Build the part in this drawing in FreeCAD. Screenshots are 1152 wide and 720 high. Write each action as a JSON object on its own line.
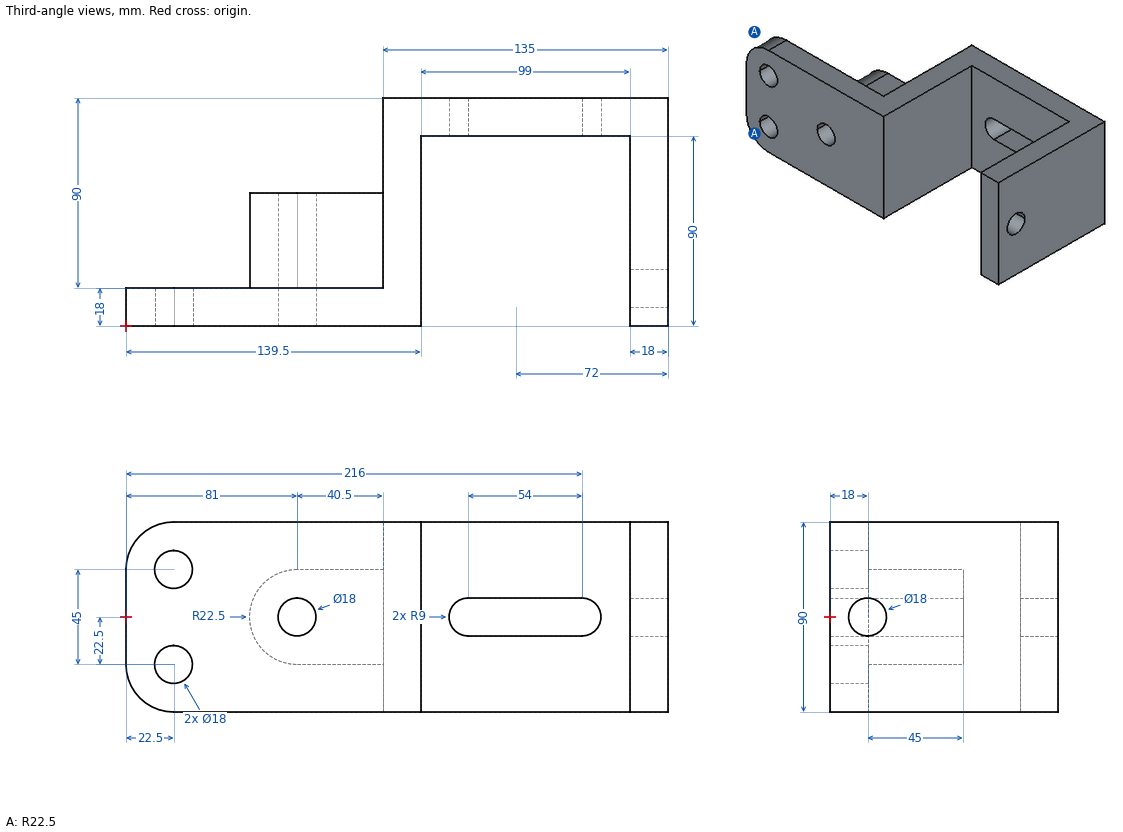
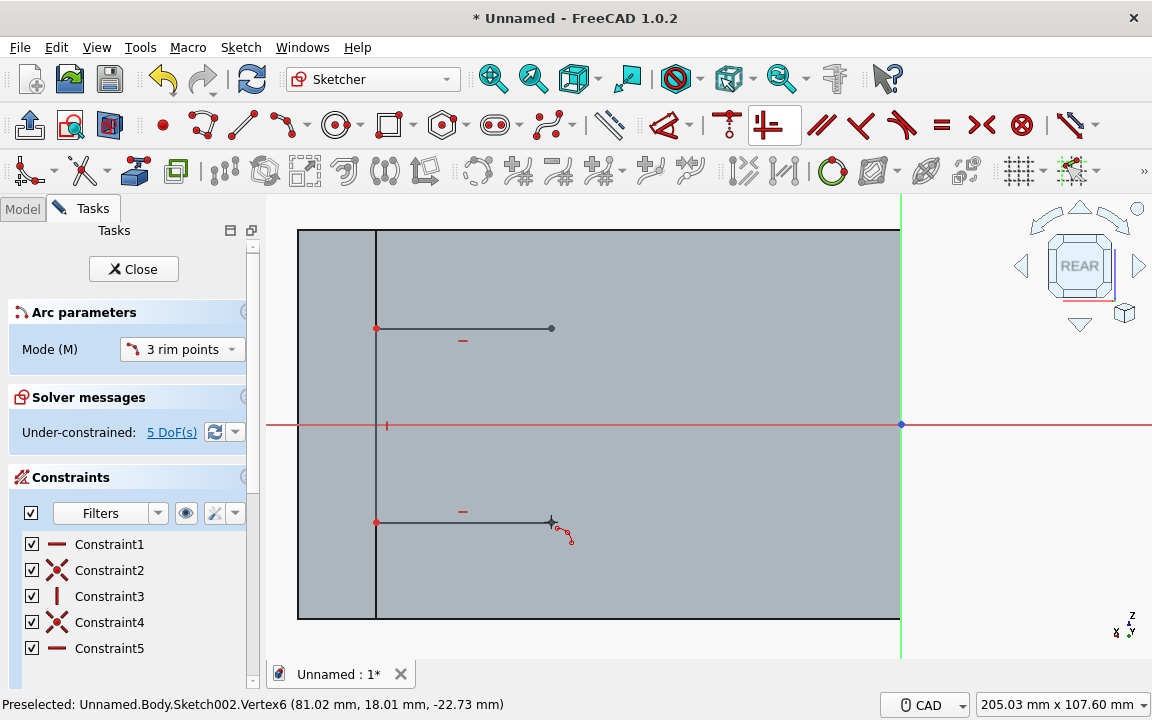
{"action": "left_click", "coordinate": [551, 523]}
{"action": "left_click", "coordinate": [551, 329]}
{"action": "left_click", "coordinate": [644, 455]}
{"action": "key", "text": "Escape"}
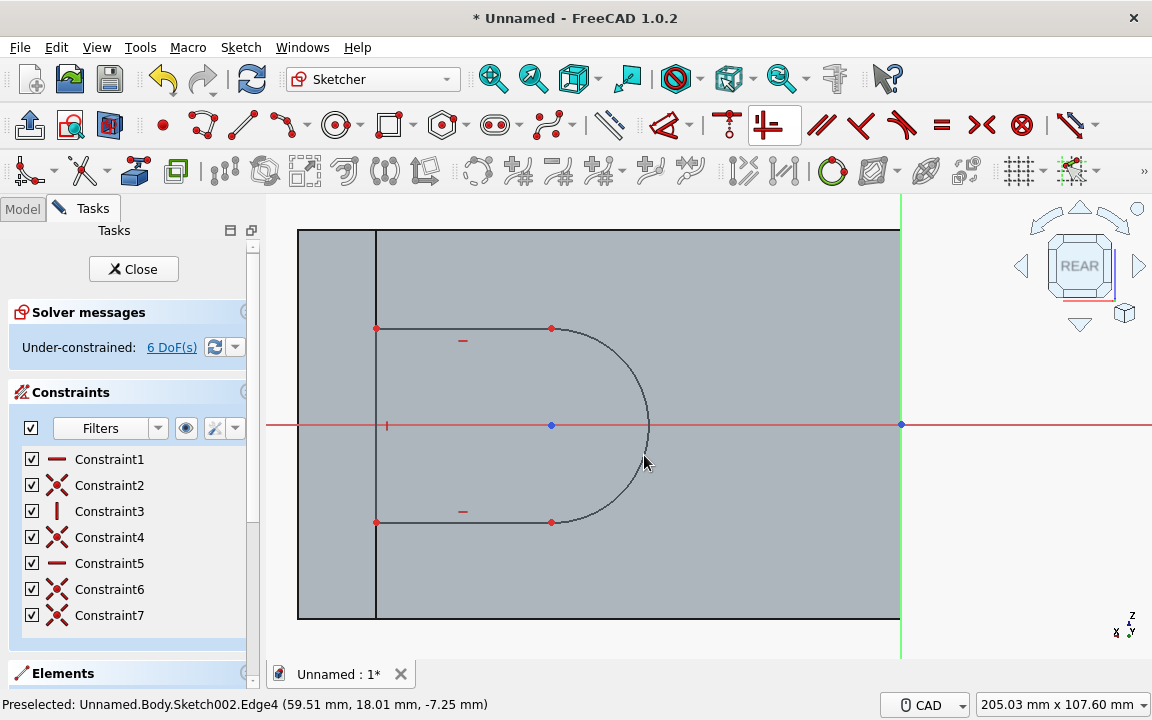
{"action": "left_click", "coordinate": [499, 329]}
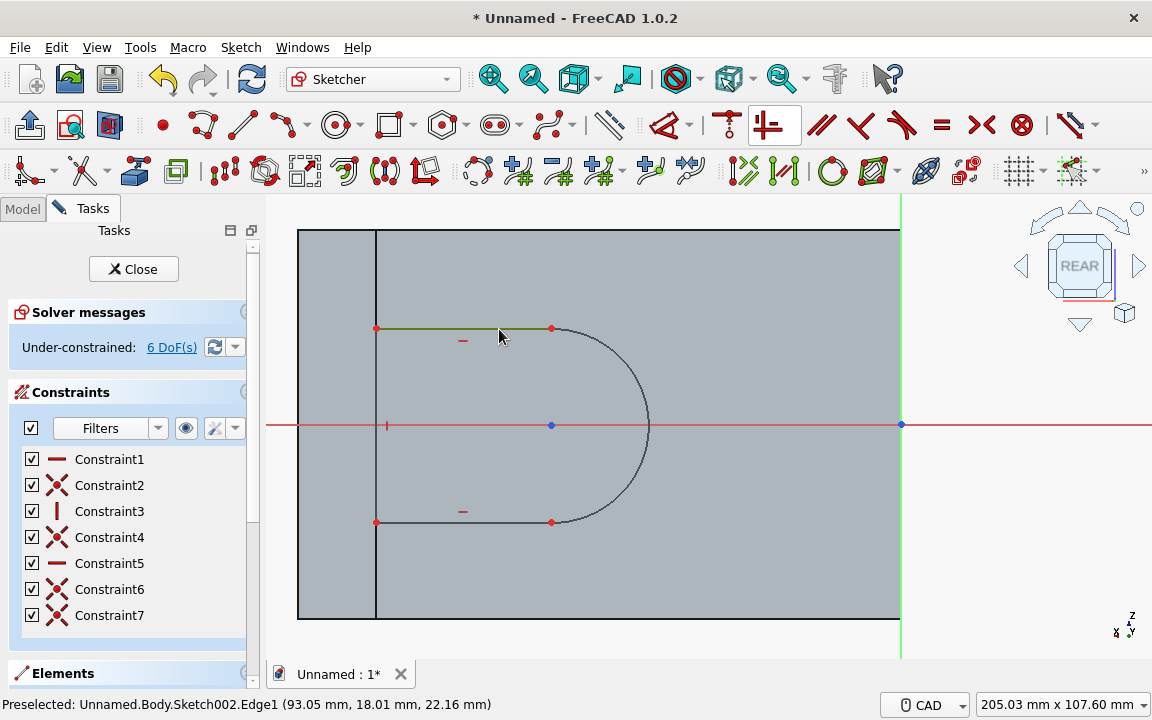
{"action": "left_click", "coordinate": [630, 483]}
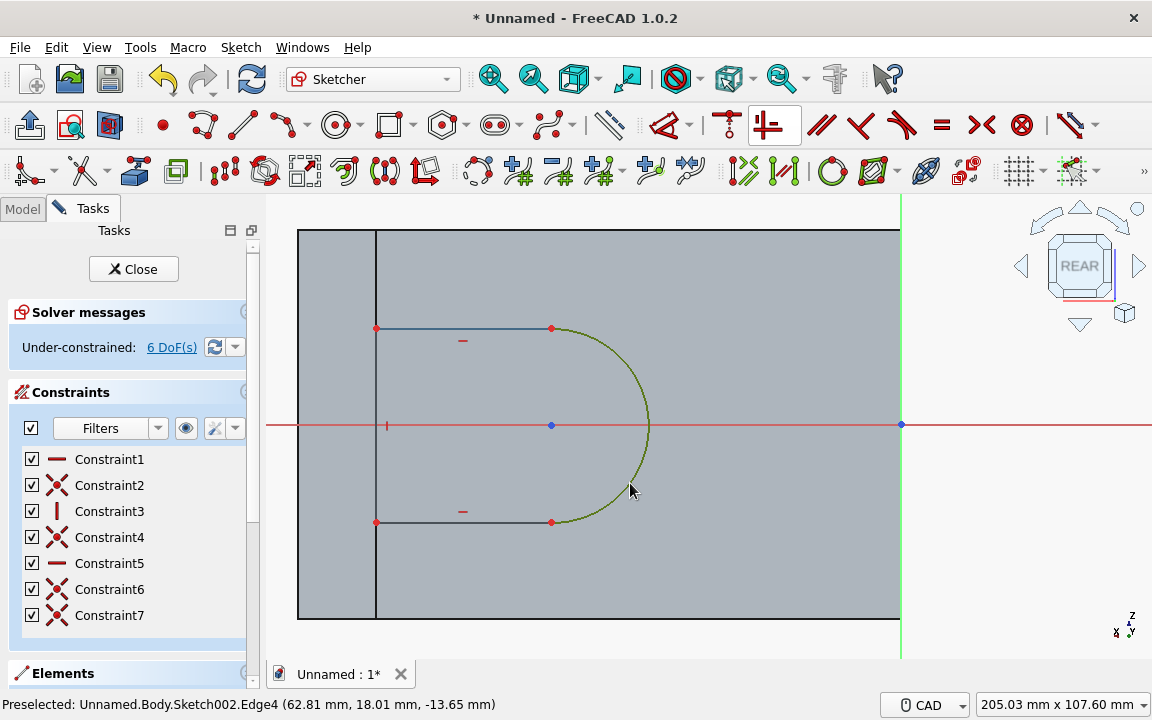
{"action": "left_click", "coordinate": [902, 126]}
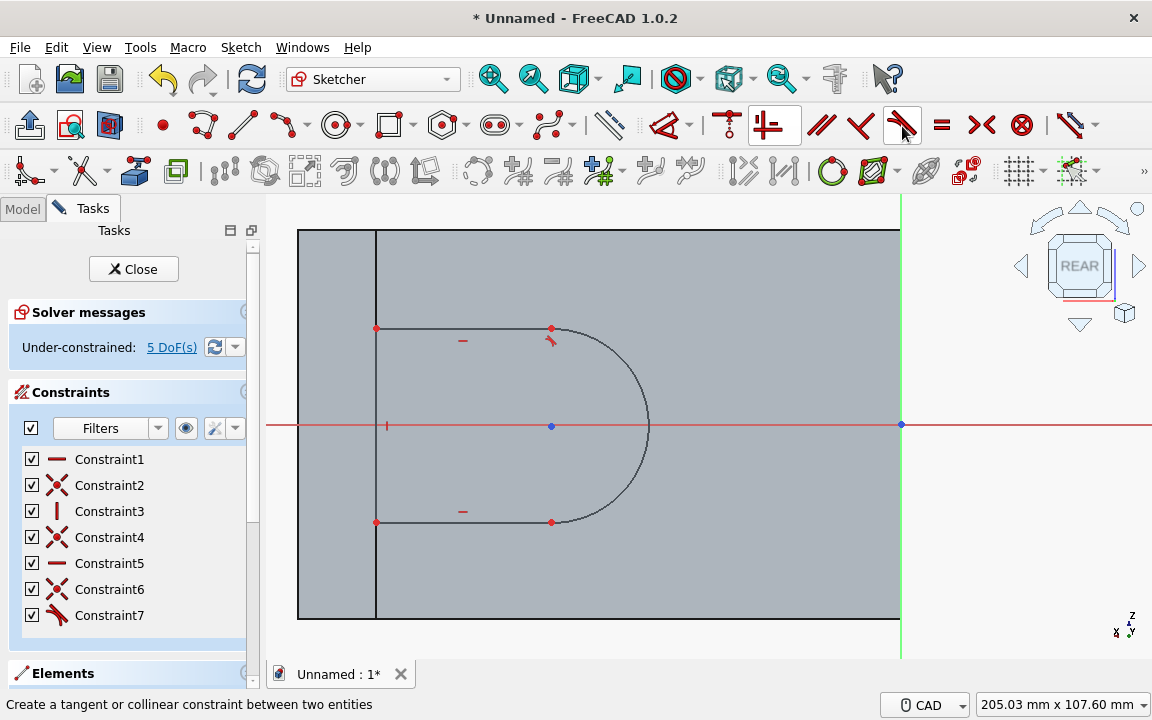
{"action": "left_click", "coordinate": [429, 523]}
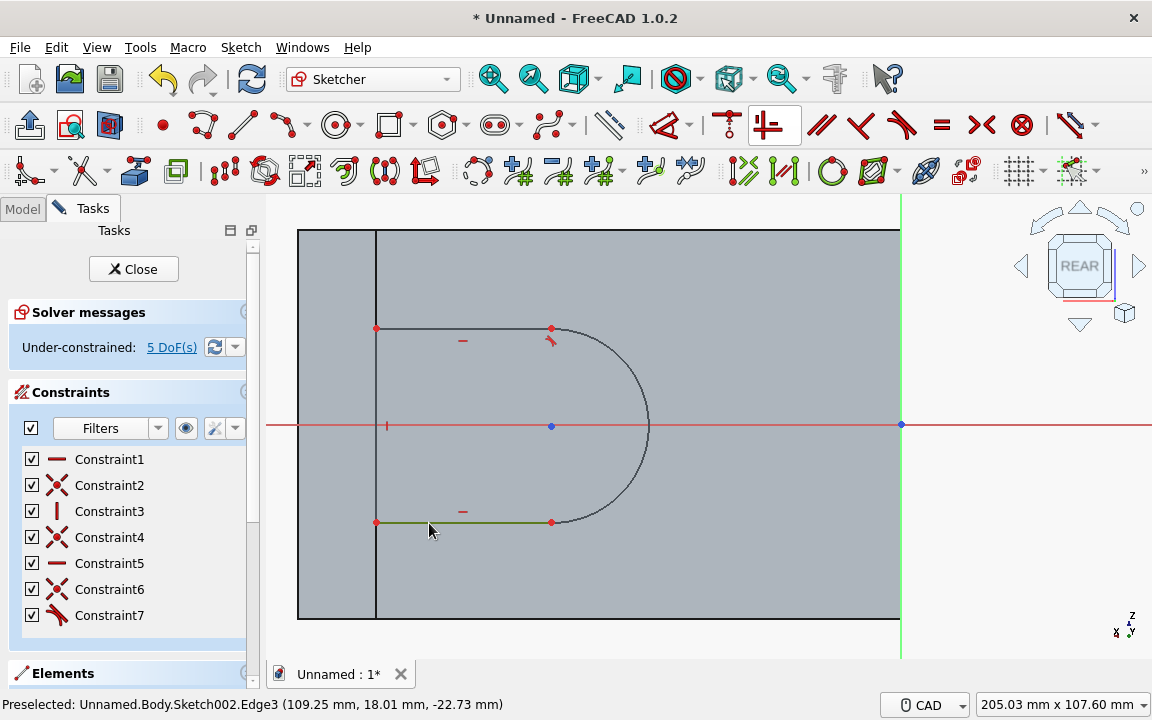
{"action": "left_click", "coordinate": [630, 483]}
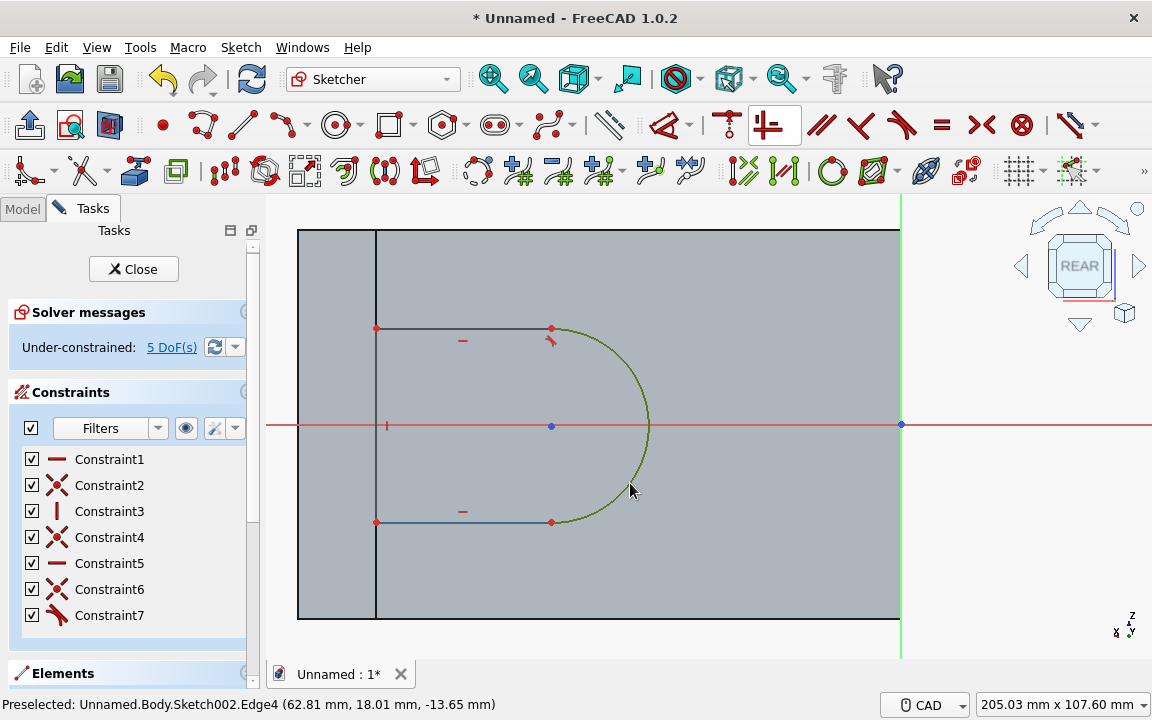
{"action": "left_click", "coordinate": [902, 126]}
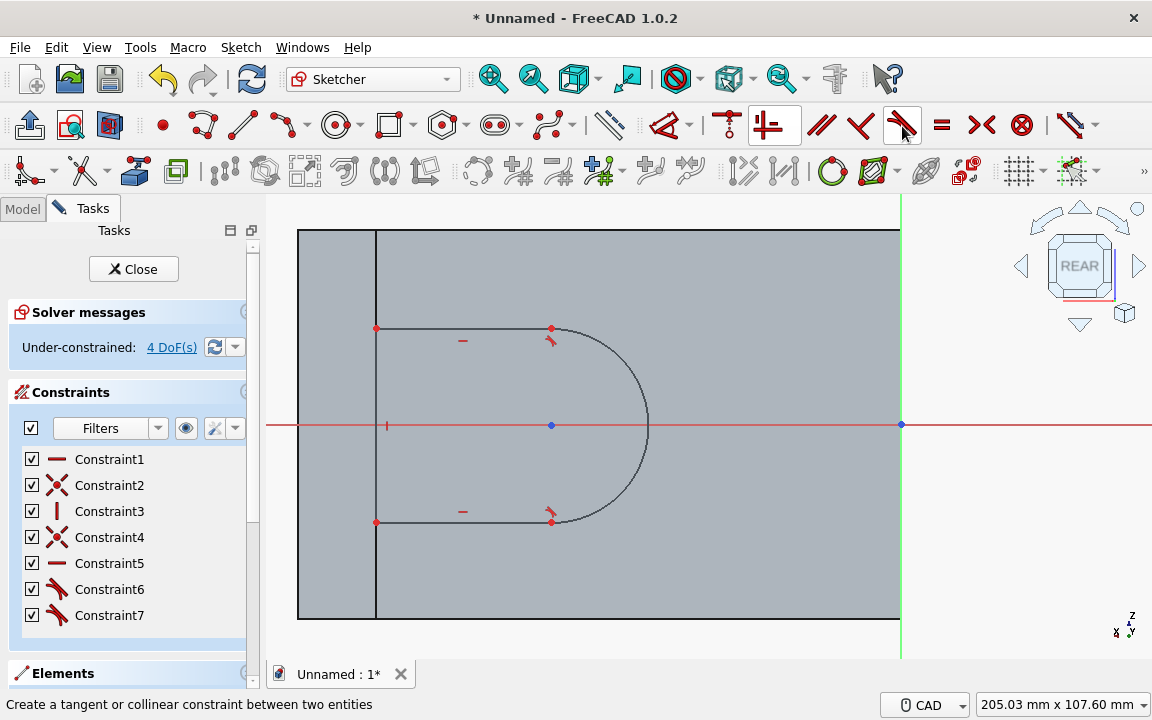
{"action": "left_click", "coordinate": [551, 426]}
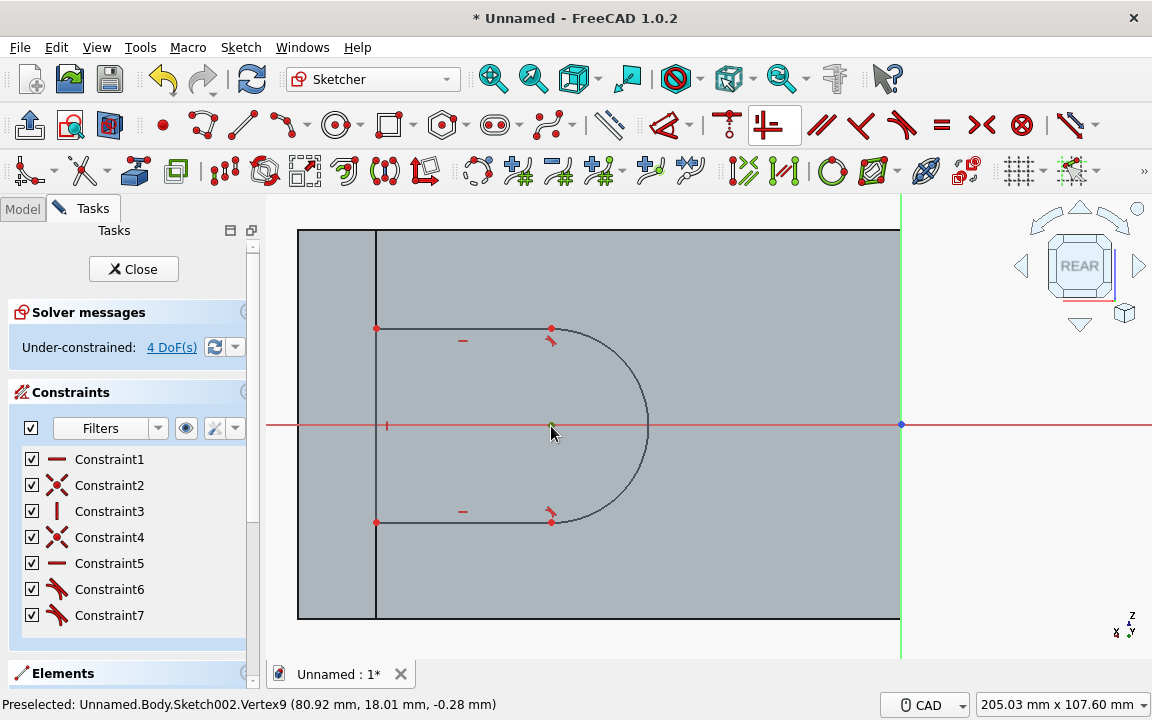
{"action": "left_click", "coordinate": [344, 425]}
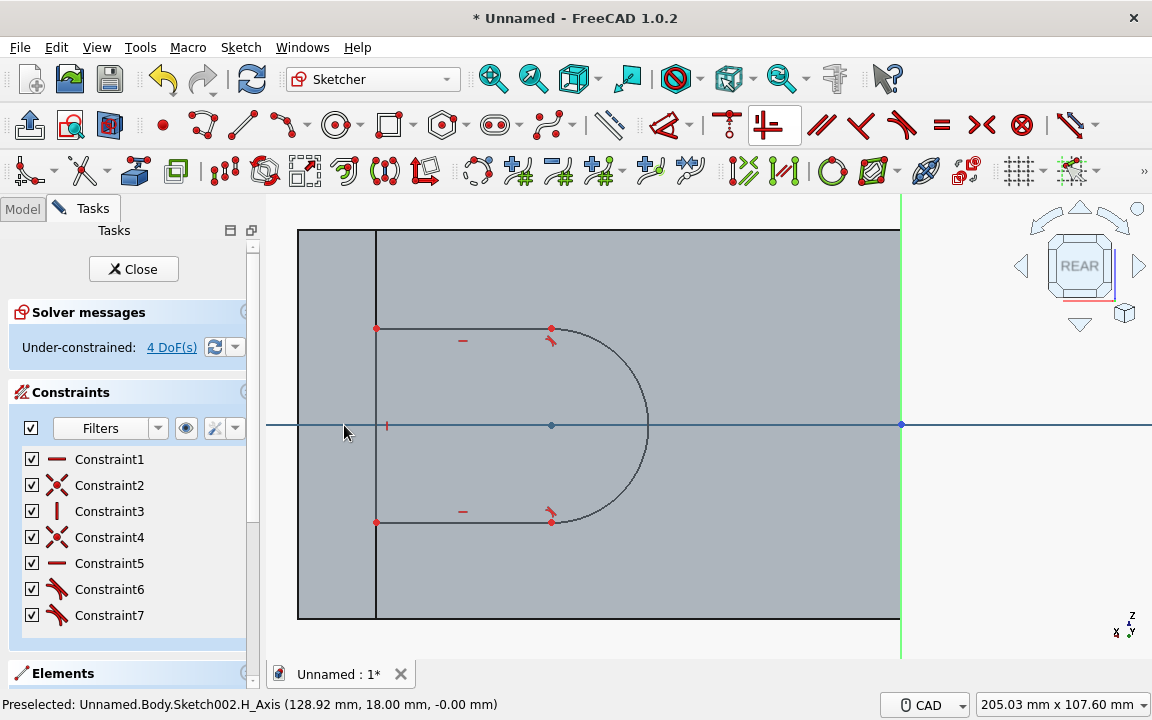
{"action": "left_click", "coordinate": [728, 126]}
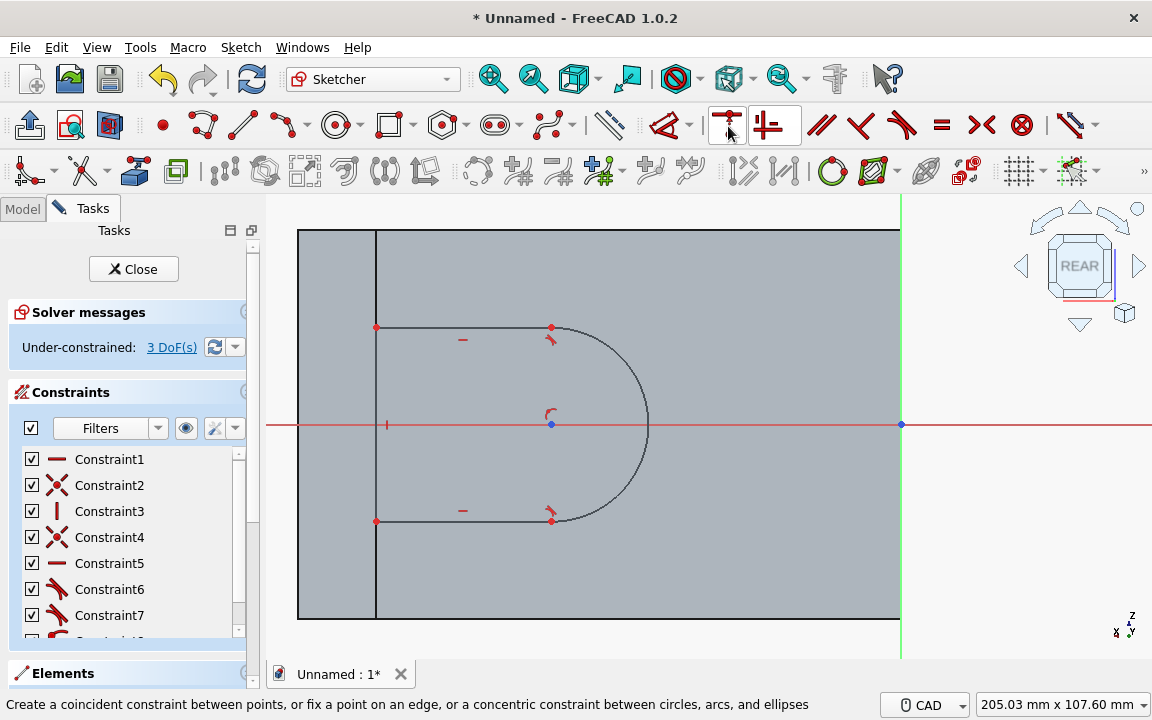
{"action": "left_click", "coordinate": [664, 126]}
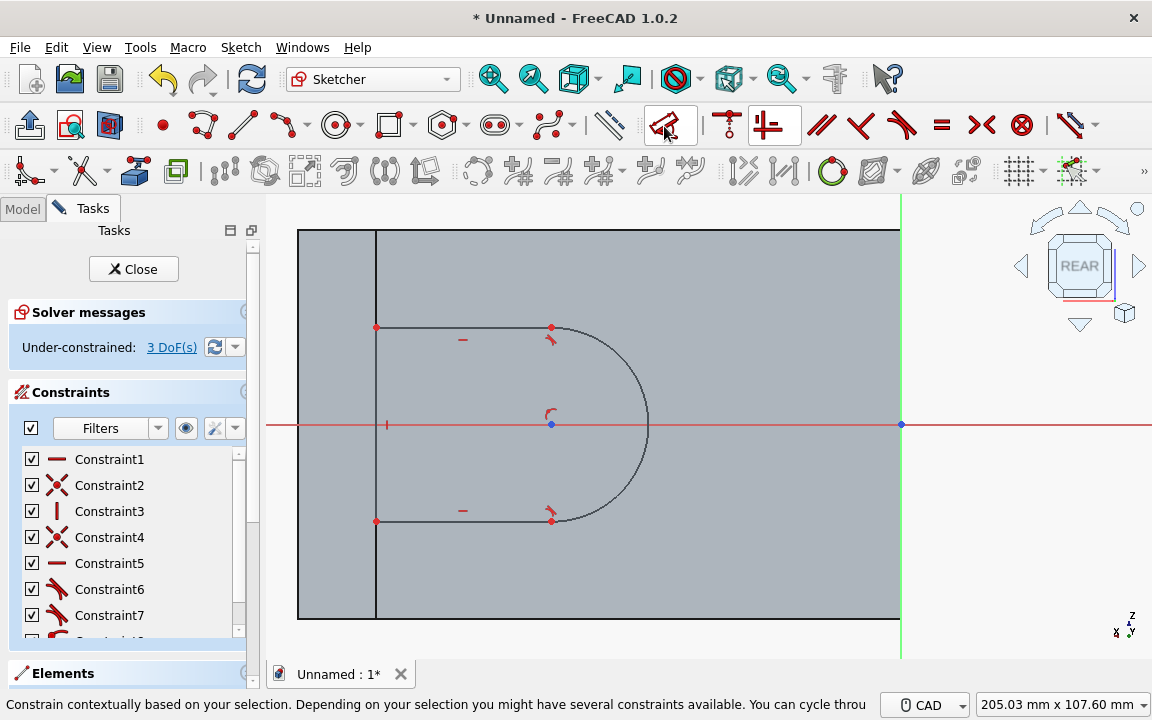
{"action": "left_click", "coordinate": [630, 482]}
{"action": "left_click", "coordinate": [656, 501]}